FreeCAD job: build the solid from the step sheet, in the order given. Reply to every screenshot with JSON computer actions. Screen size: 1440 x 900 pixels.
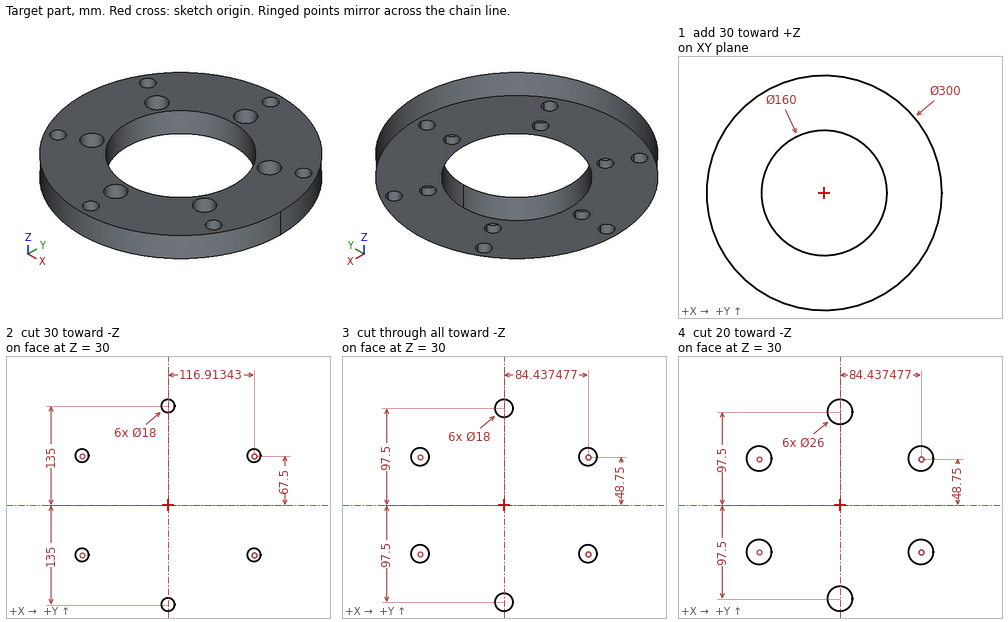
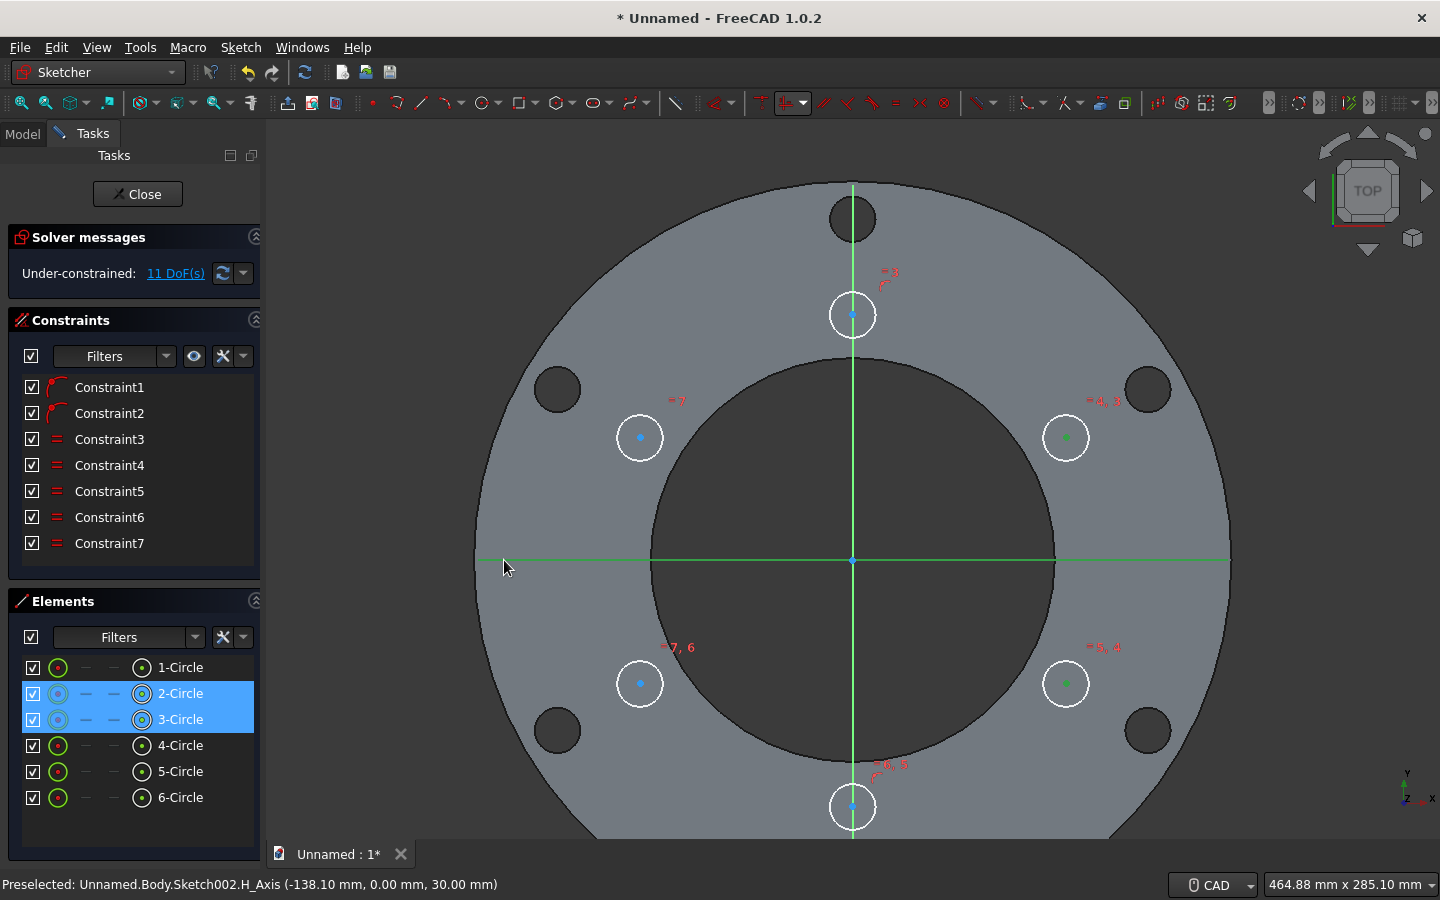
{"action": "key", "text": "s"}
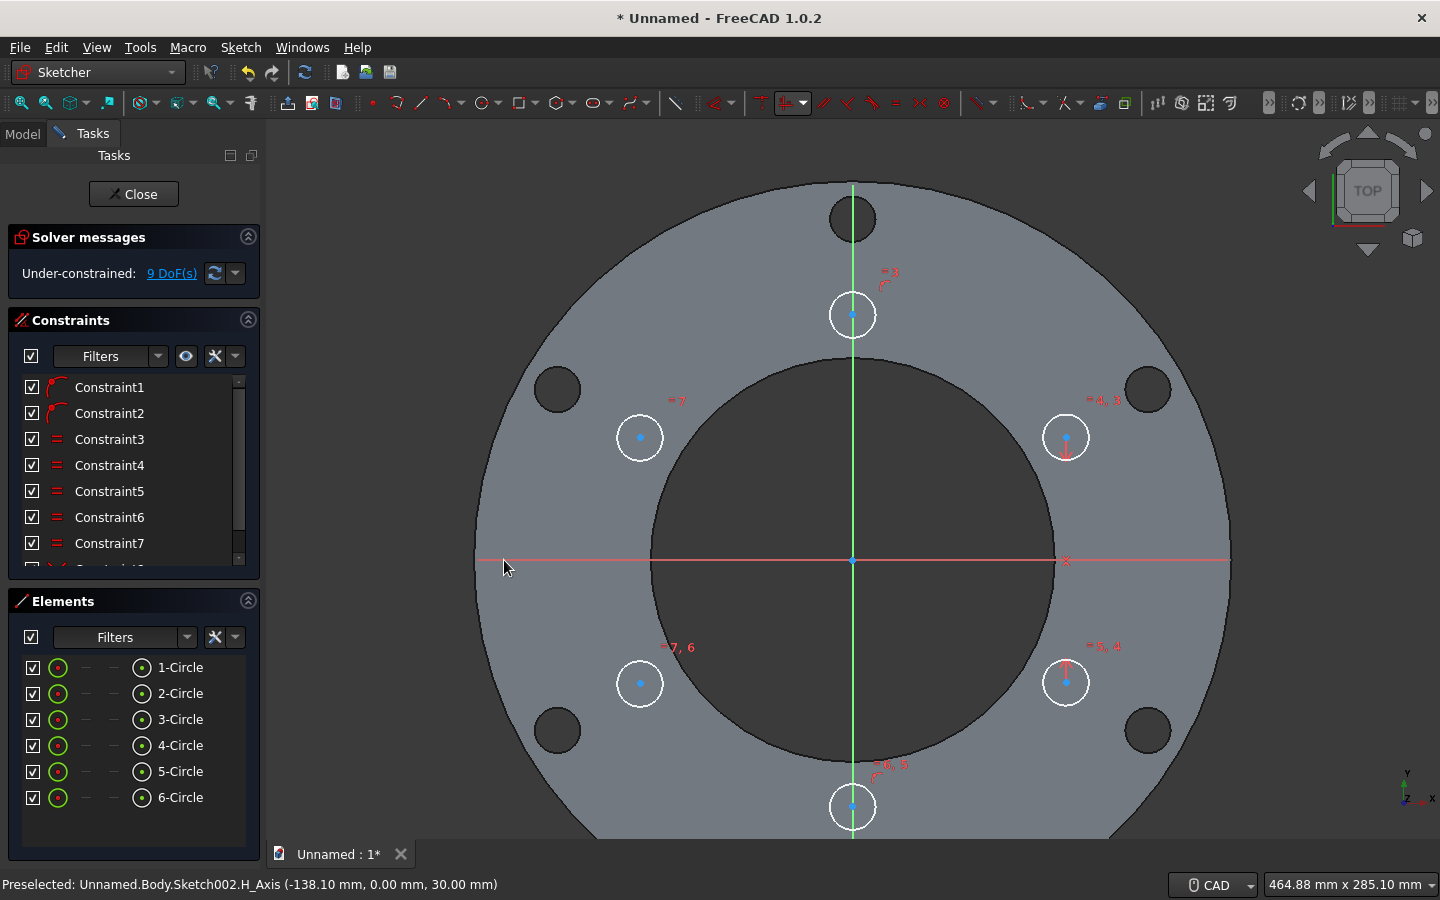
{"action": "left_click", "coordinate": [1066, 683]}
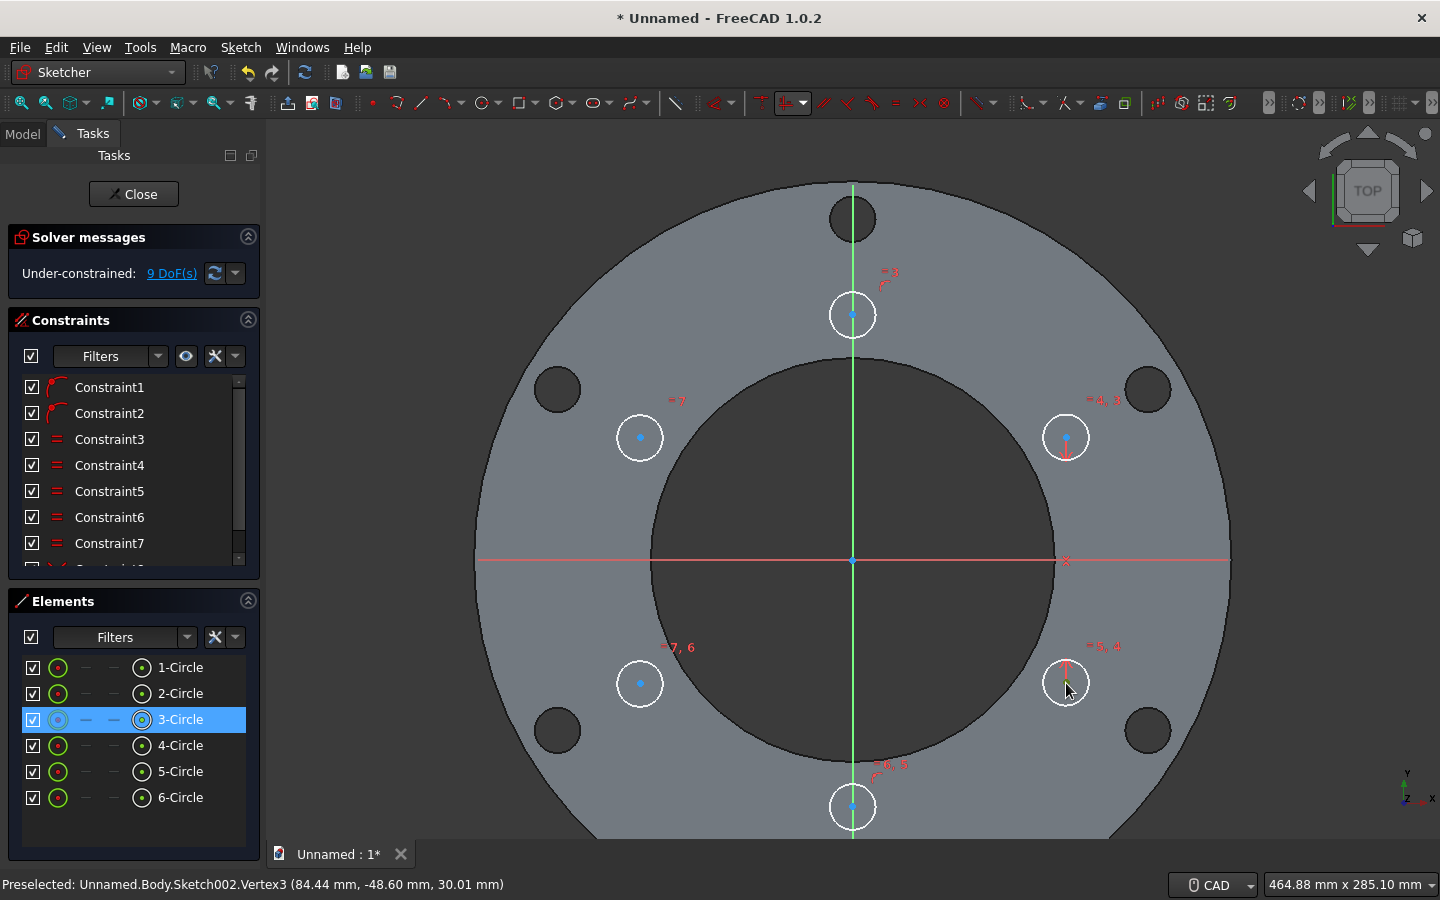
{"action": "left_click", "coordinate": [640, 684]}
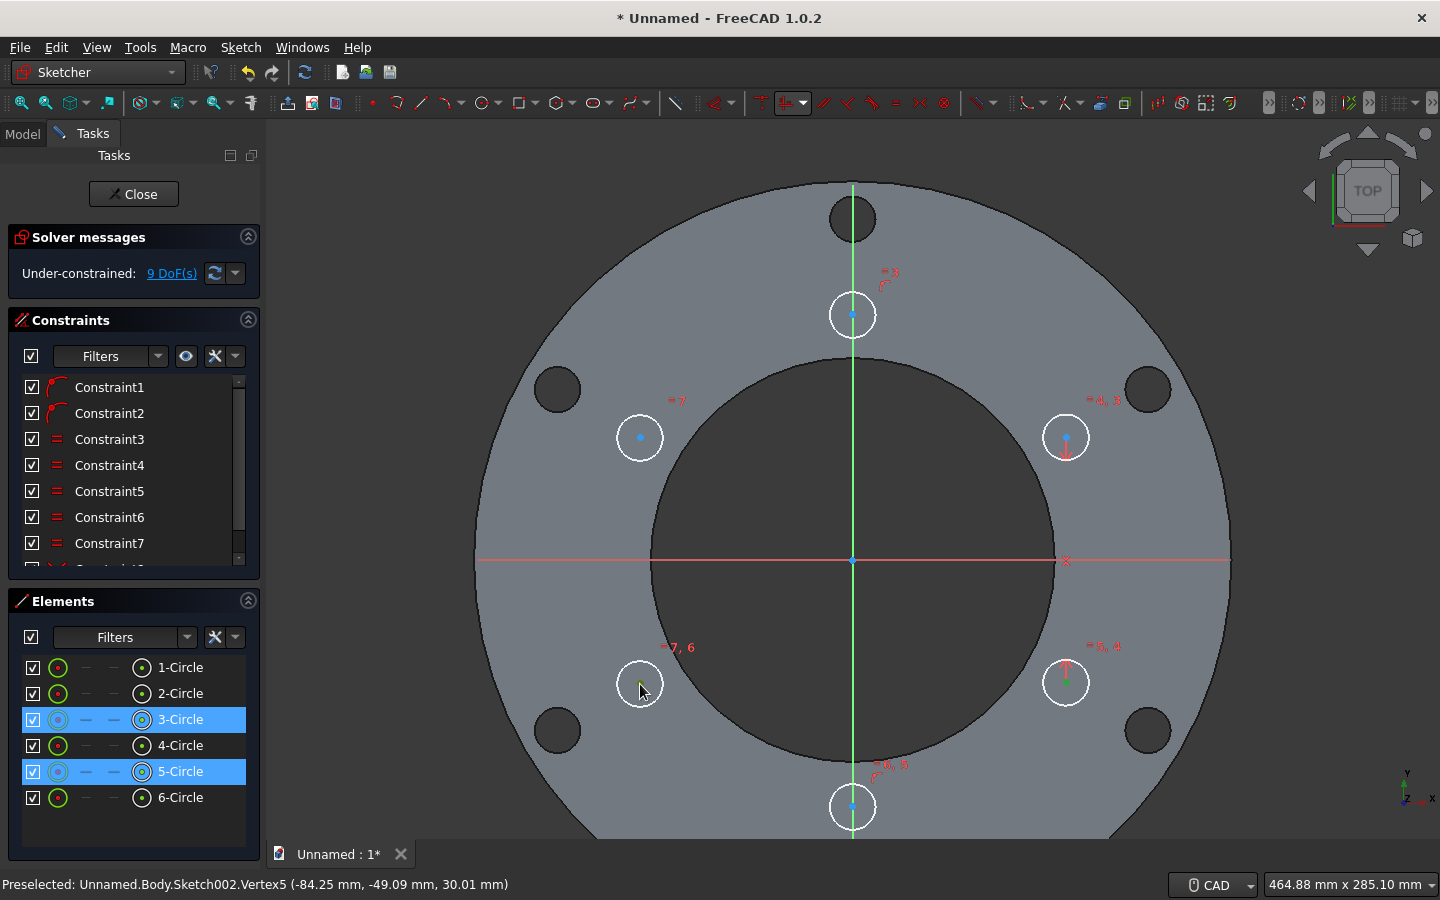
{"action": "left_click", "coordinate": [853, 716]}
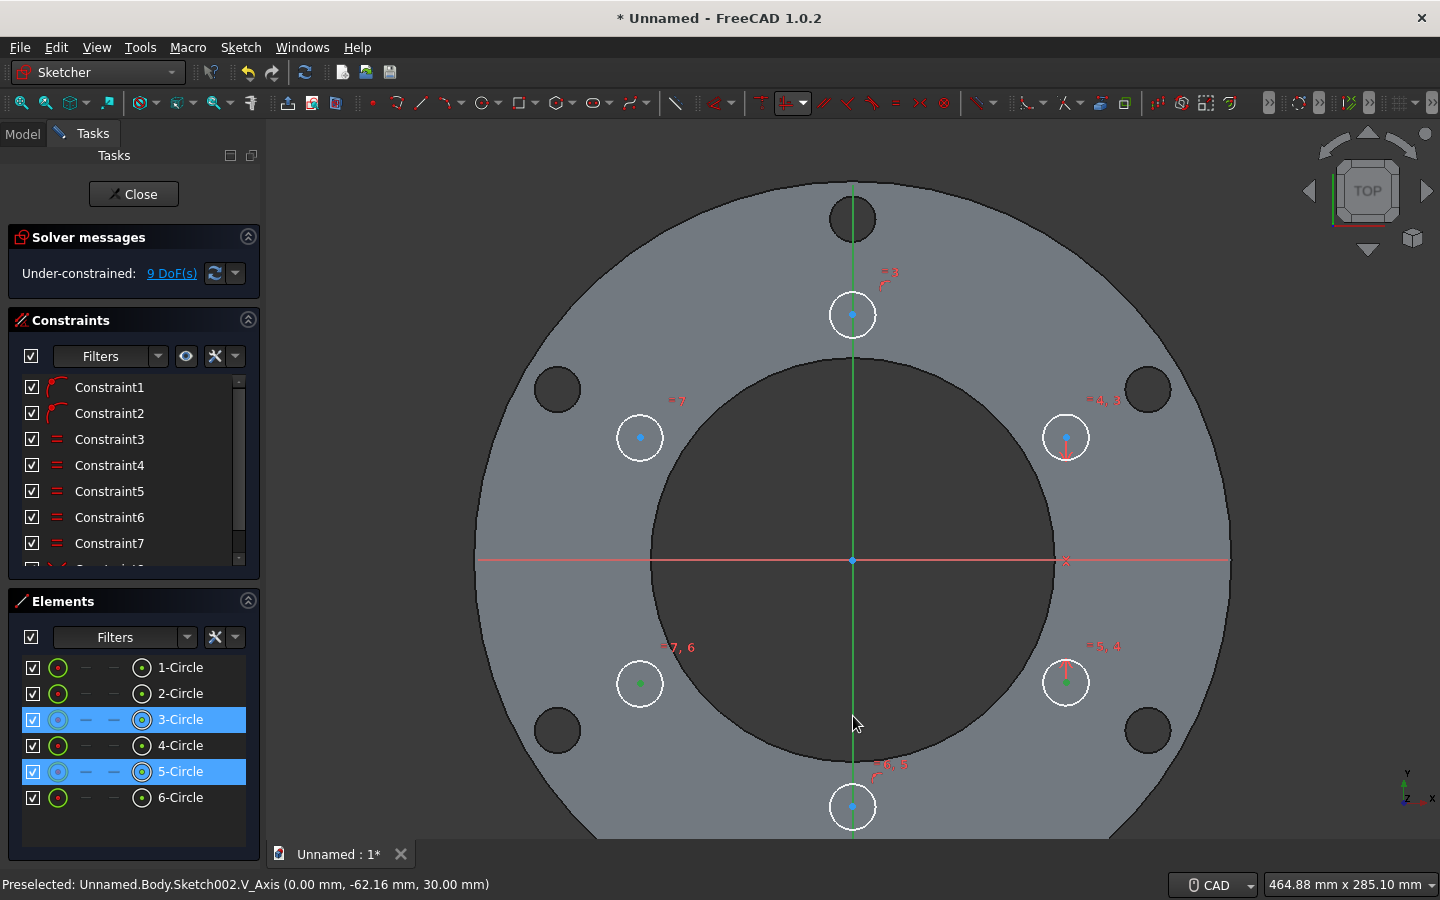
{"action": "key", "text": "s"}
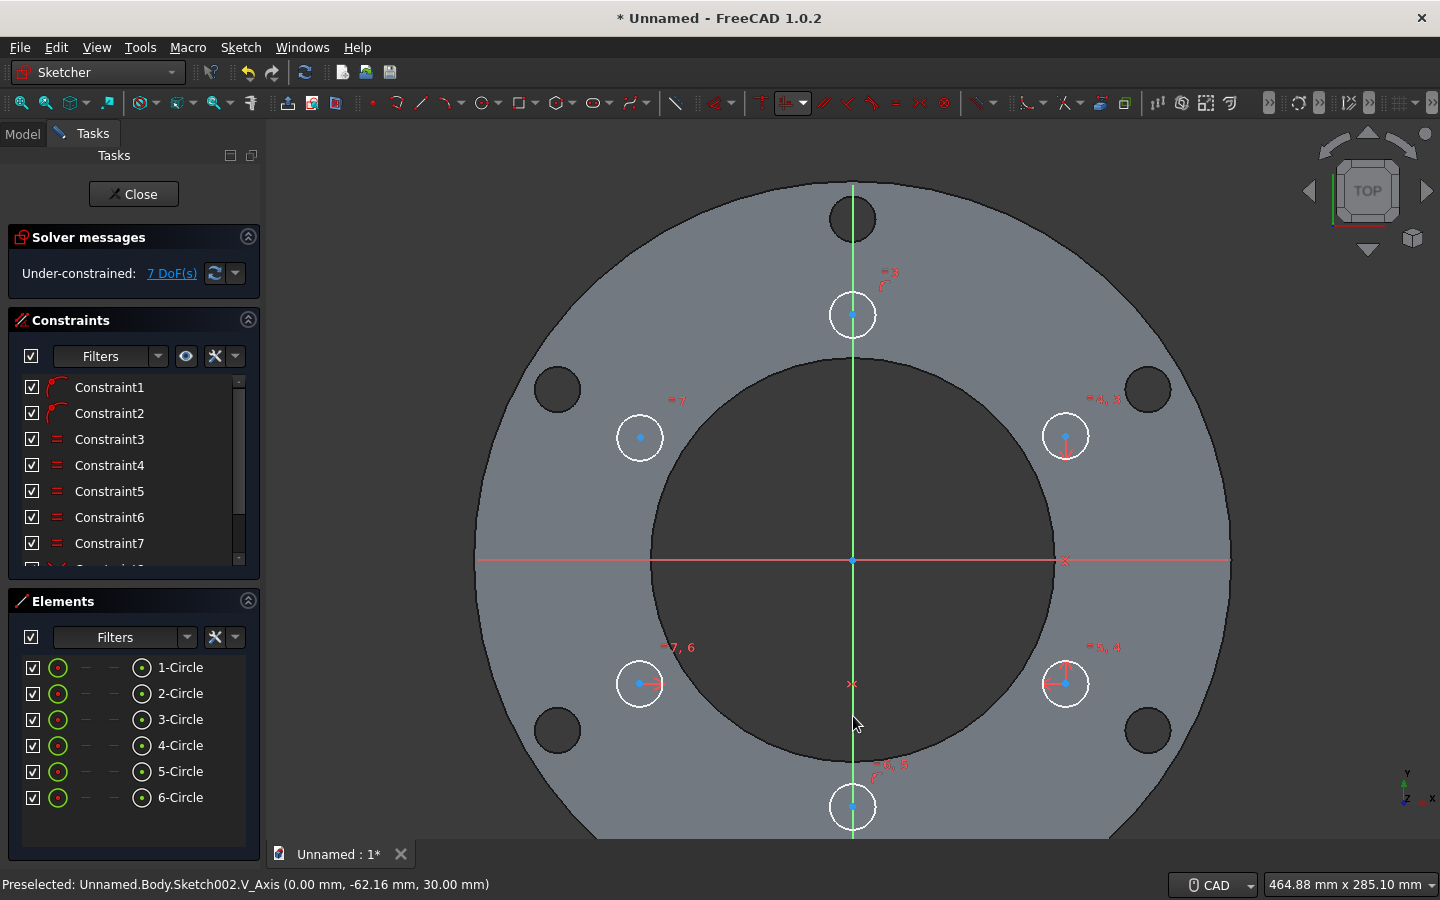
{"action": "left_click", "coordinate": [1066, 436]}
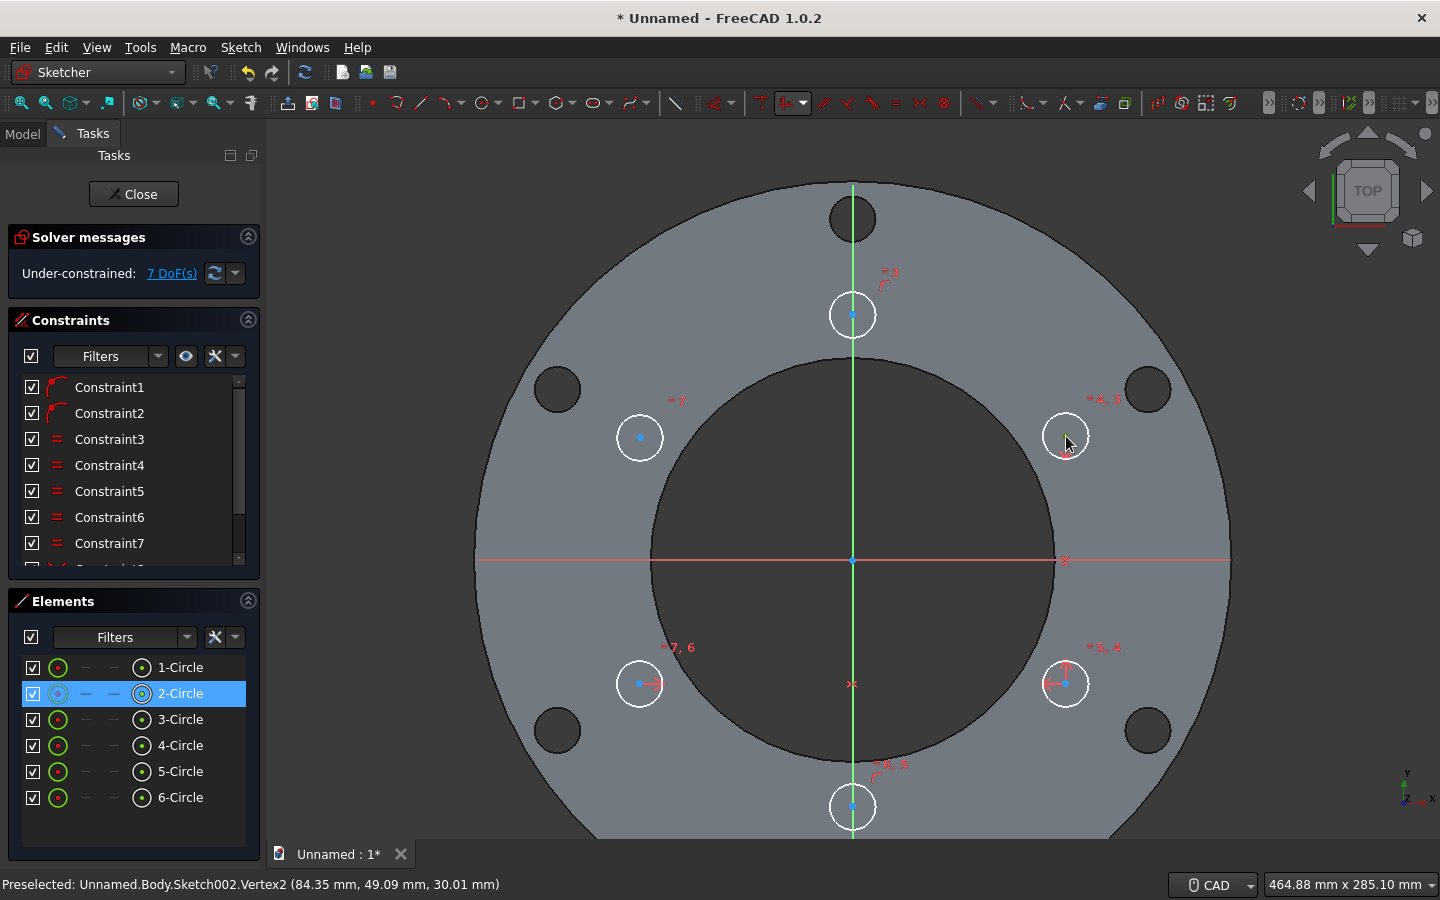
{"action": "left_click", "coordinate": [640, 438]}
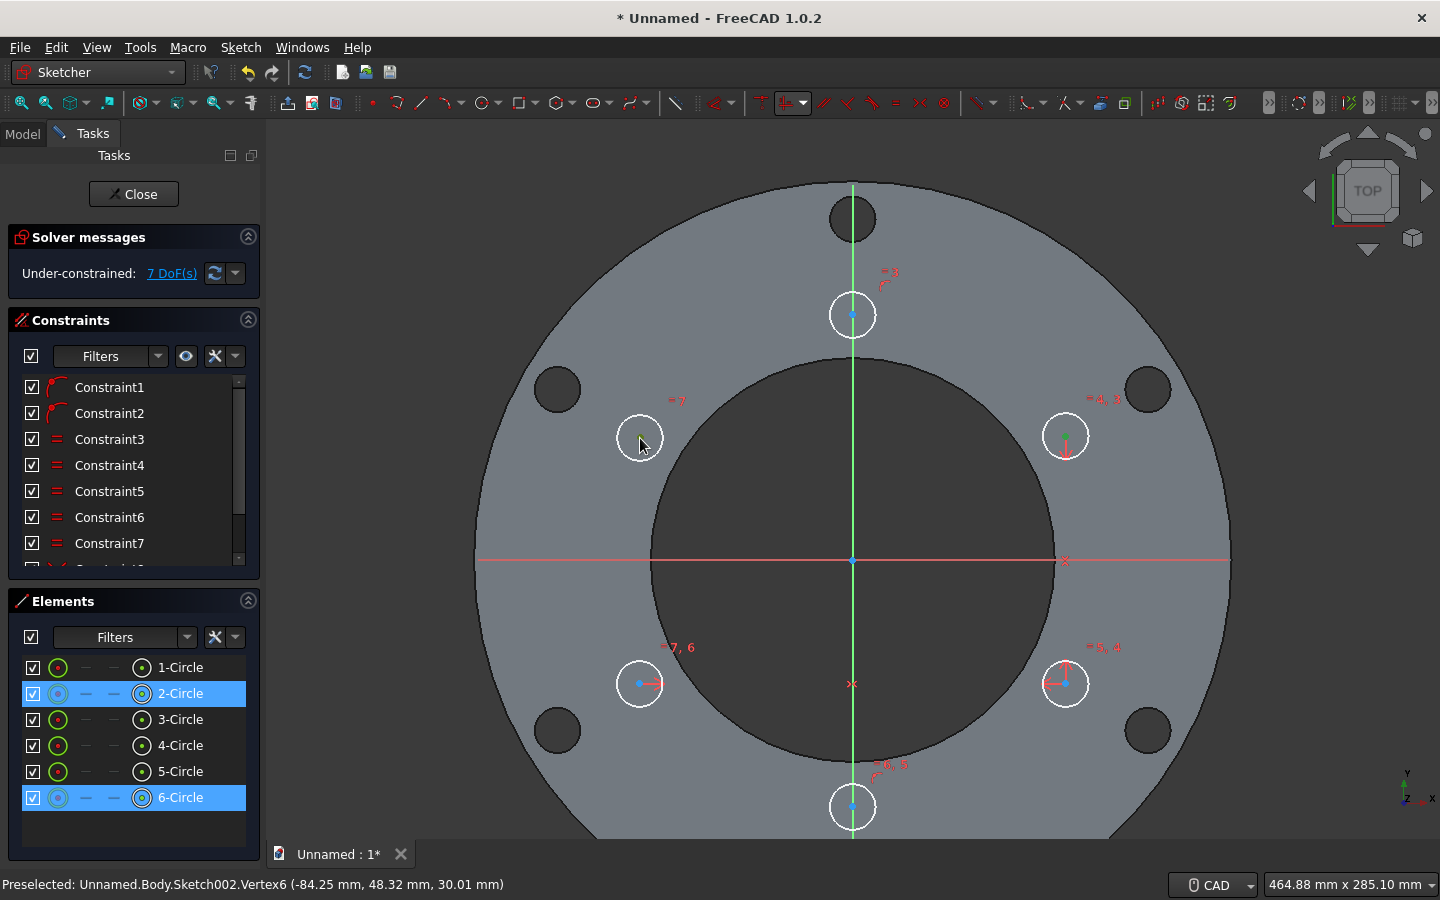
{"action": "left_click", "coordinate": [853, 716]}